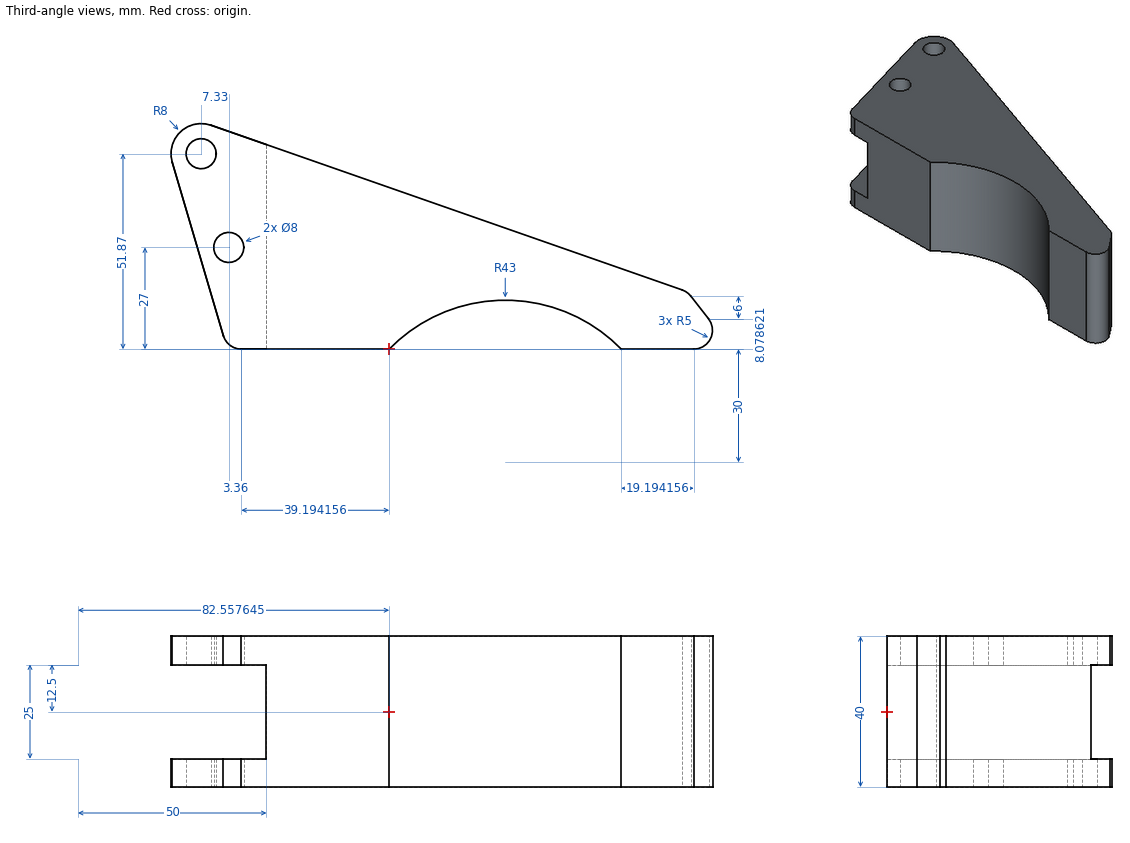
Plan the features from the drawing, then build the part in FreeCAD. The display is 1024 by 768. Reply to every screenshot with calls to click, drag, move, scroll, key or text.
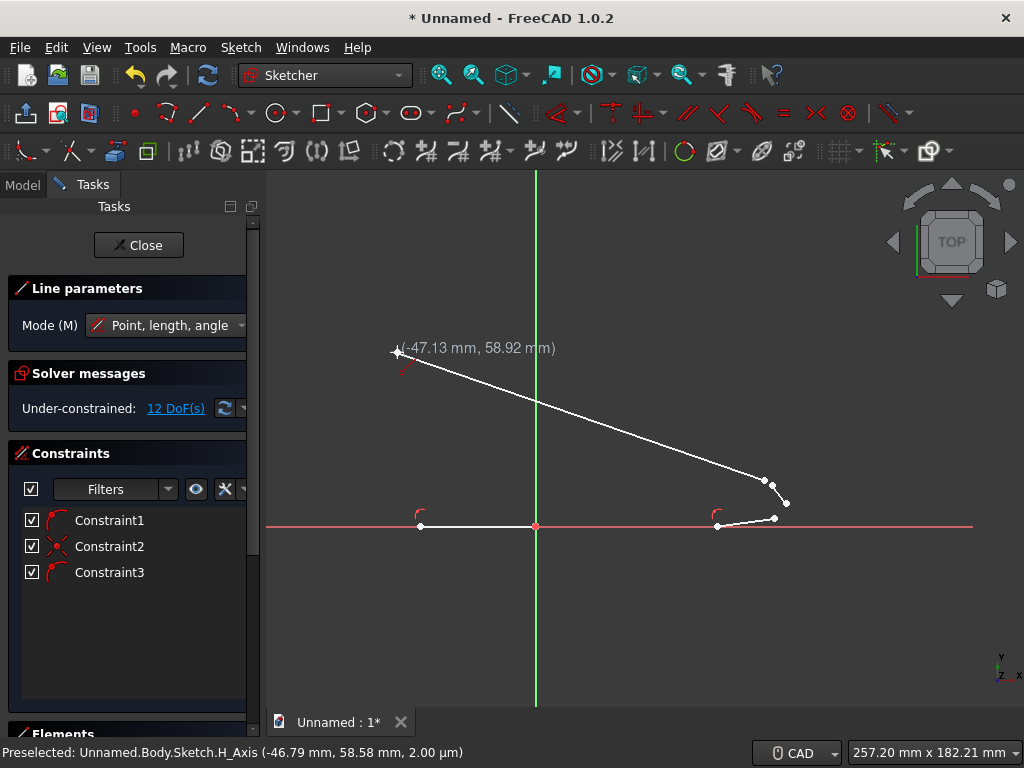
click(366, 380)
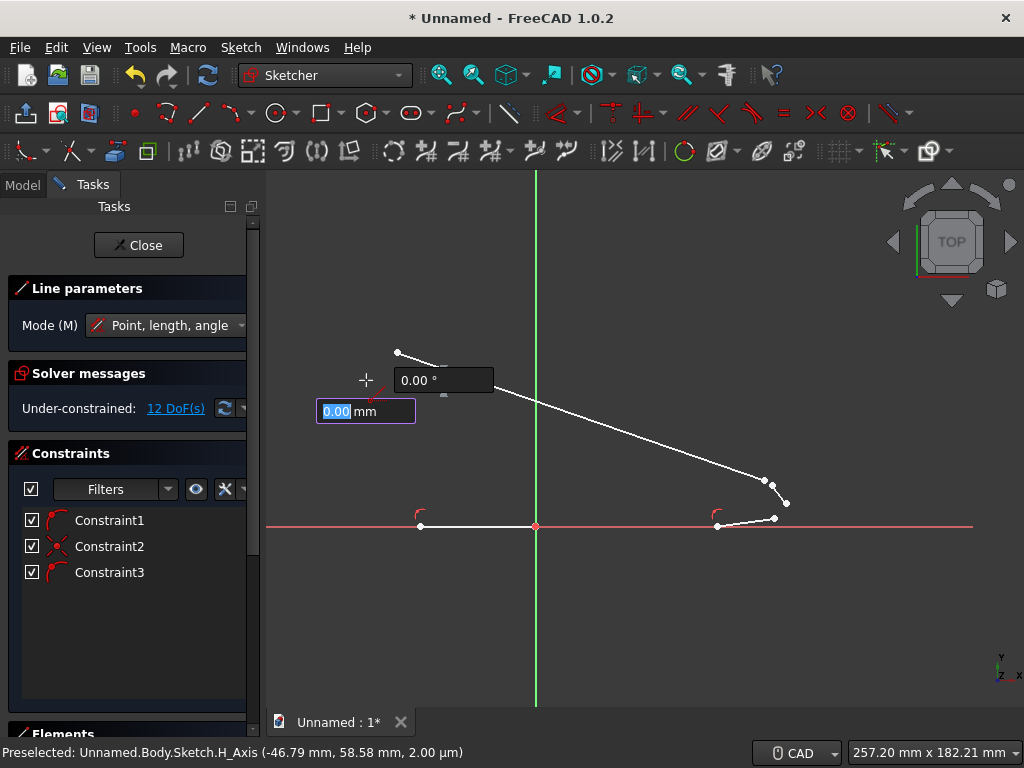
scroll(406, 516, up, 3)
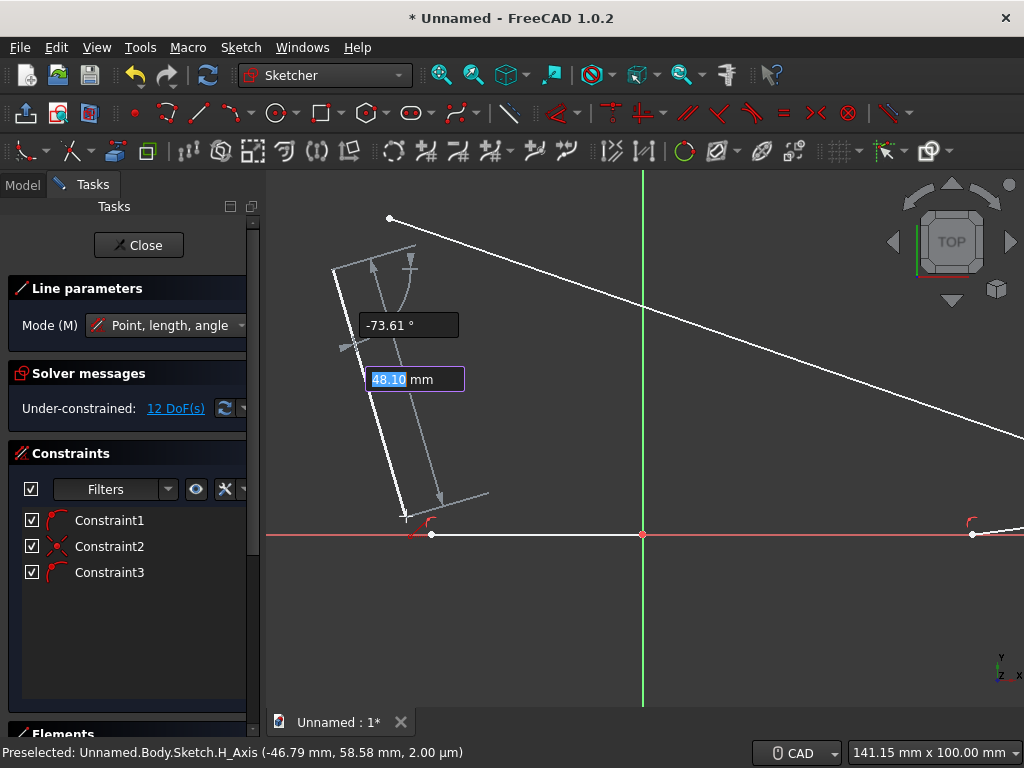
click(406, 516)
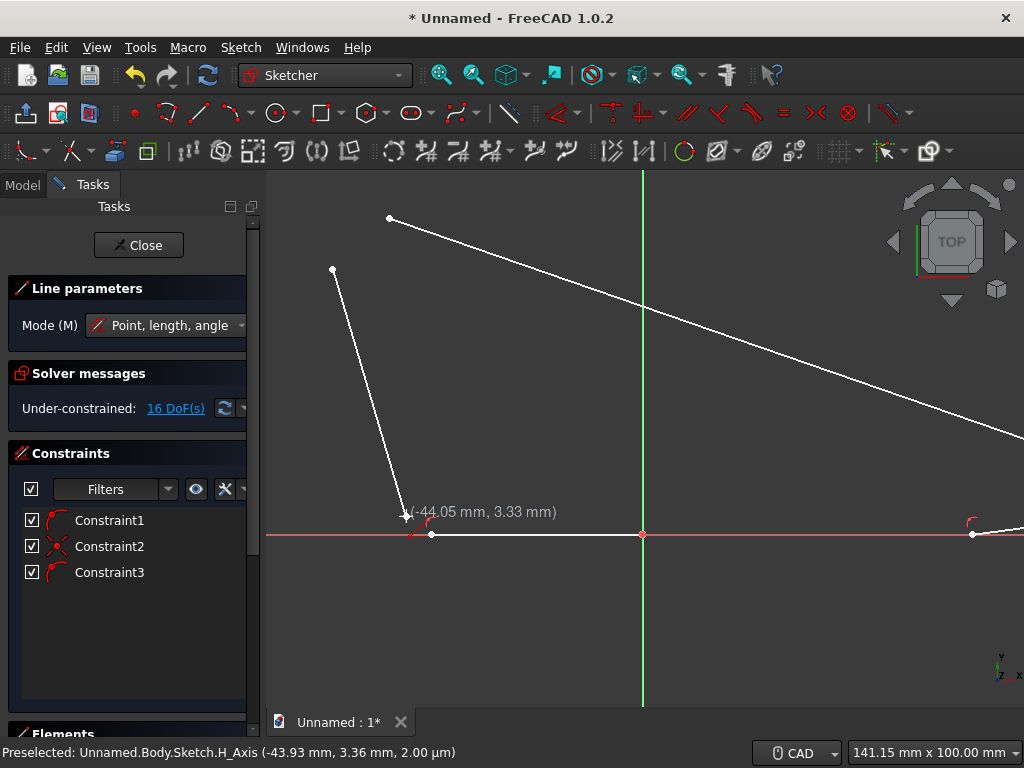
click(232, 114)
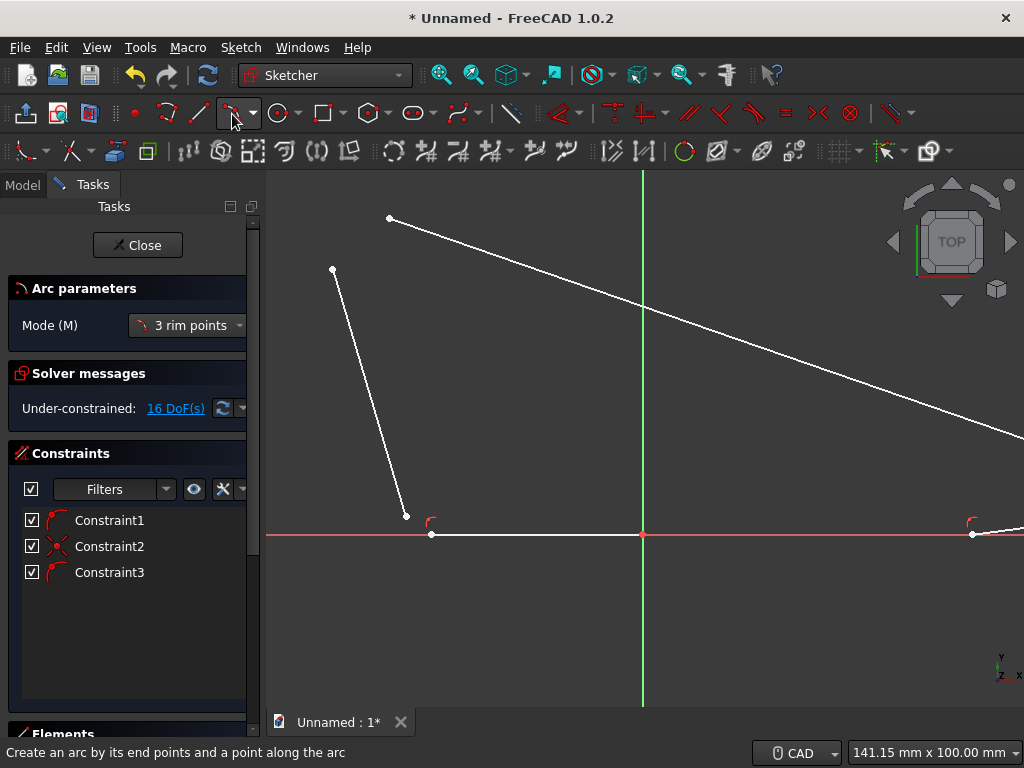
click(643, 535)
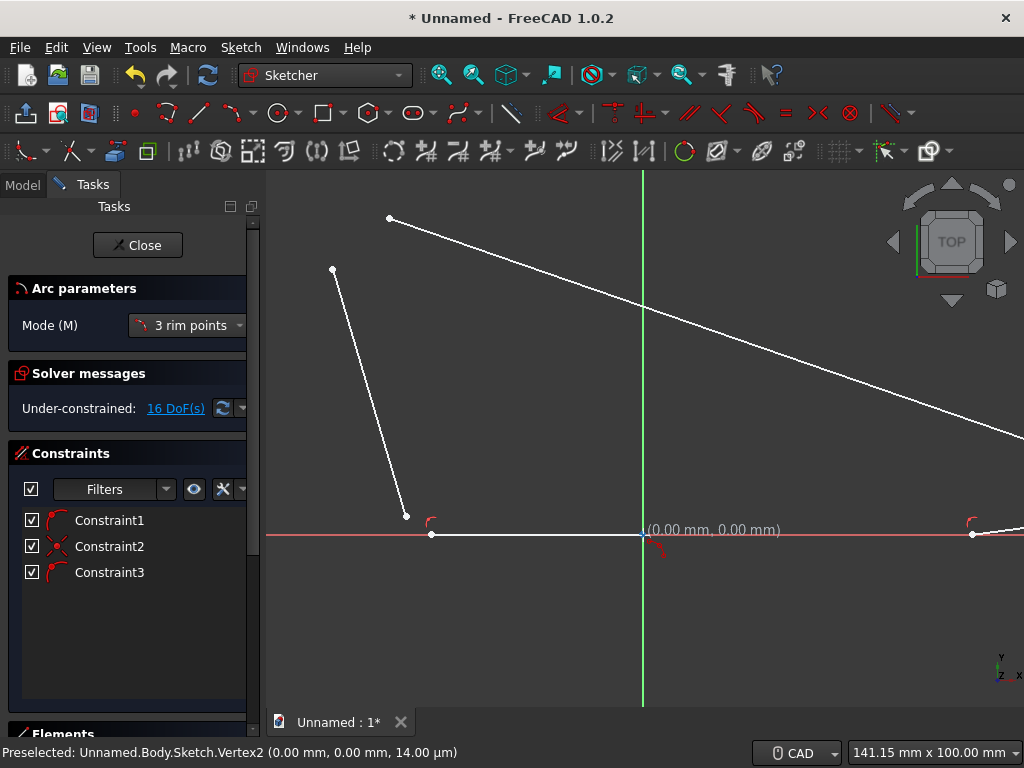
scroll(406, 515, down, 3)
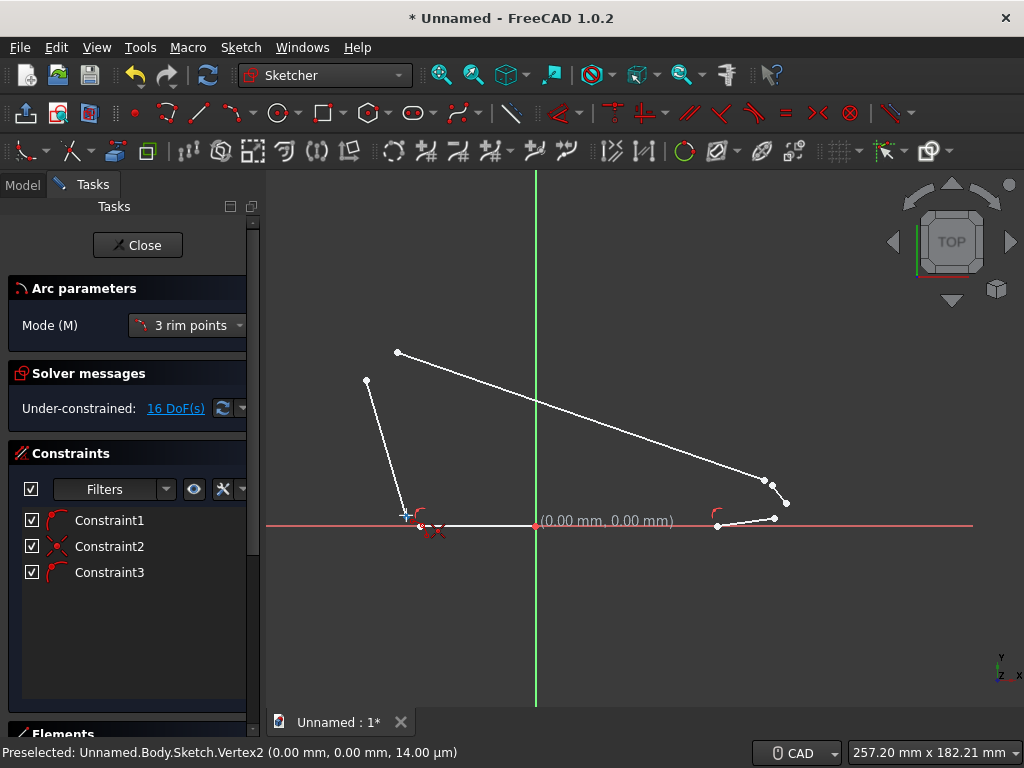
click(717, 526)
click(627, 488)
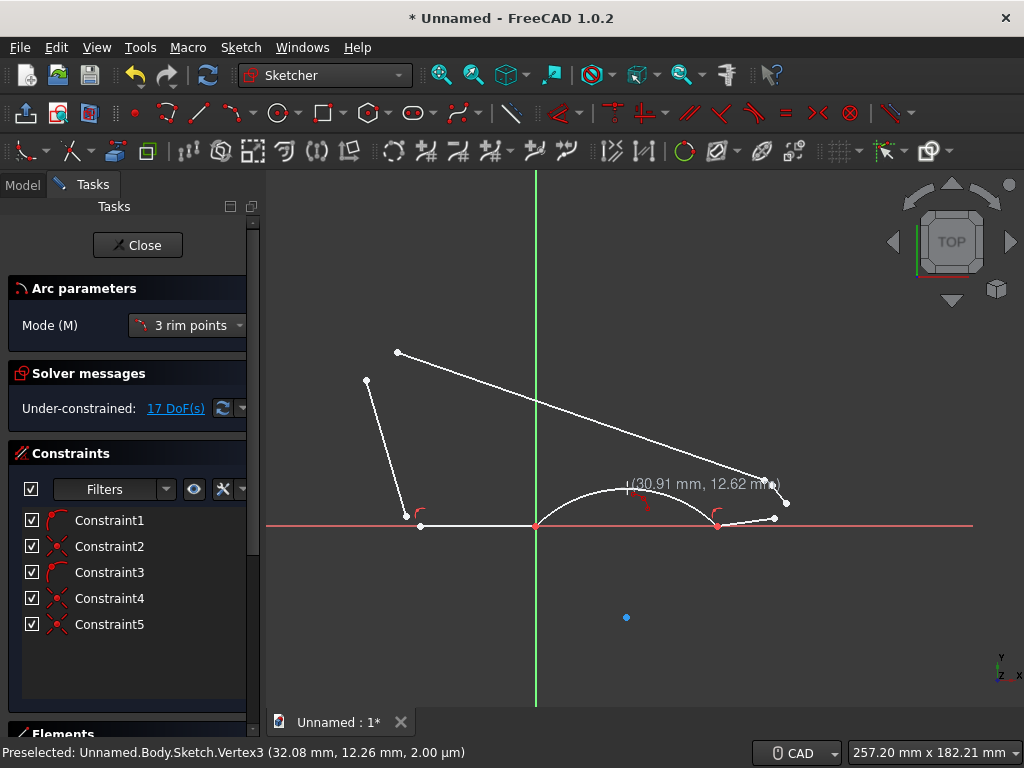
click(774, 519)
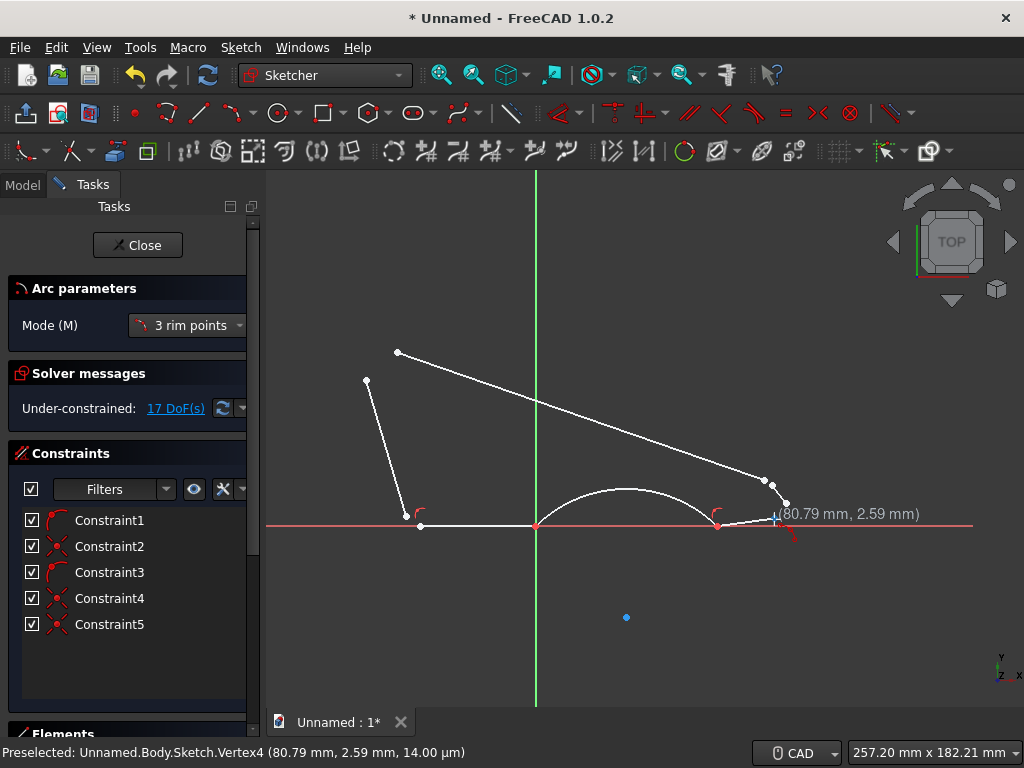
scroll(786, 502, up, 2)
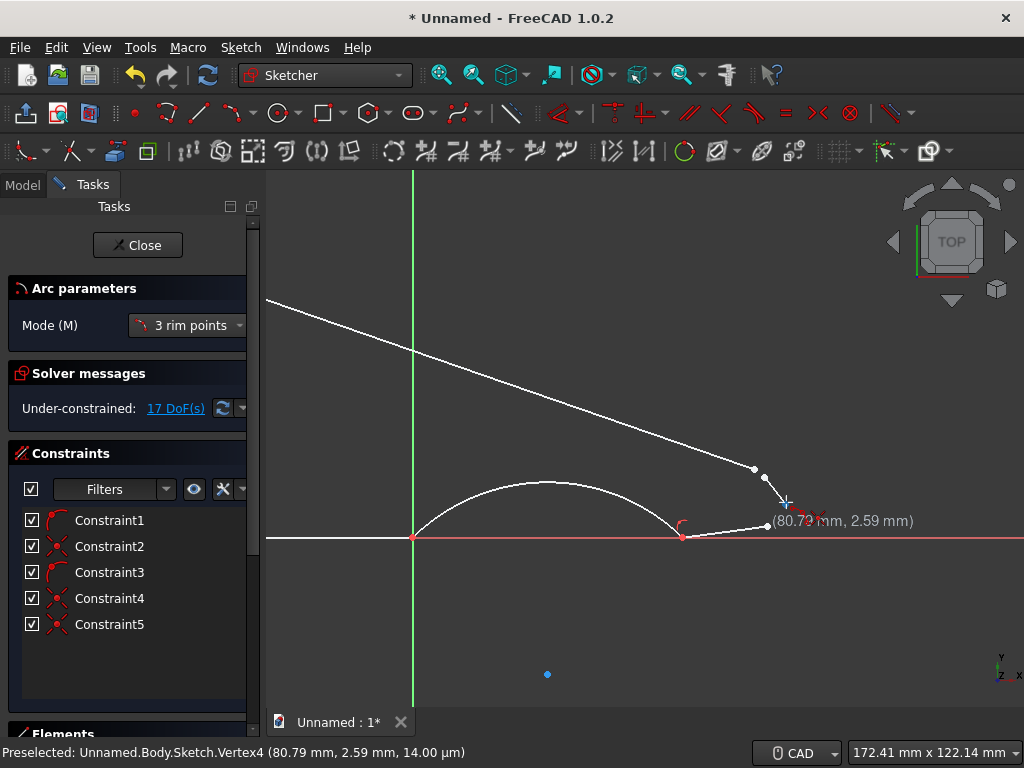
click(786, 504)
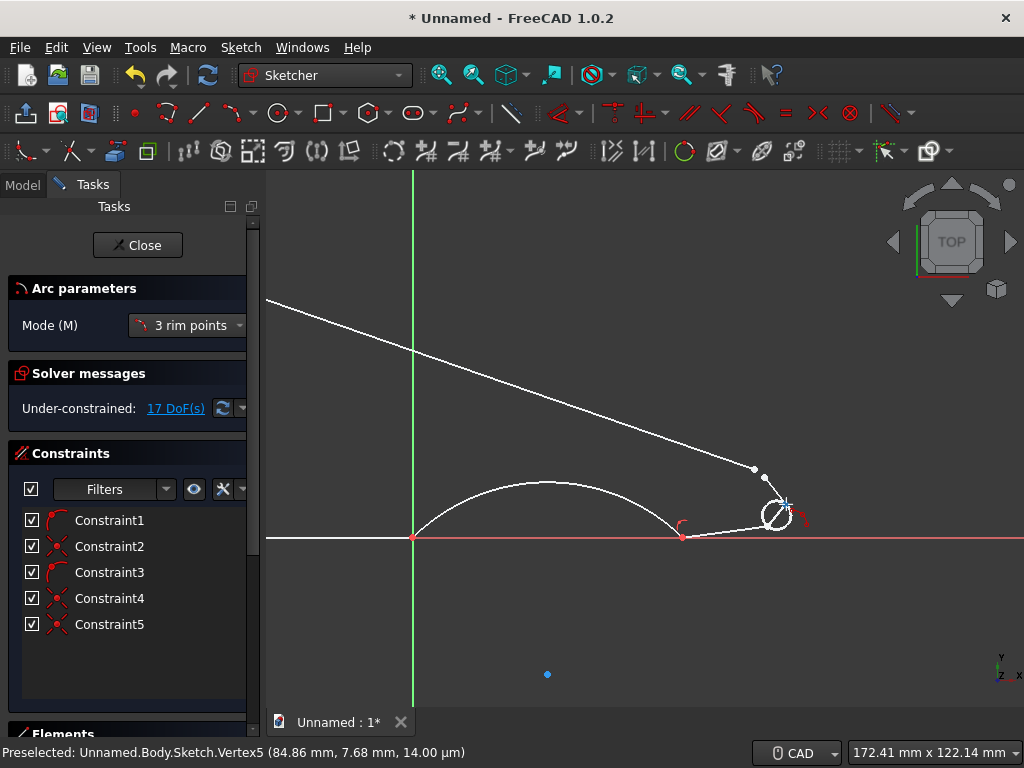
scroll(788, 525, up, 2)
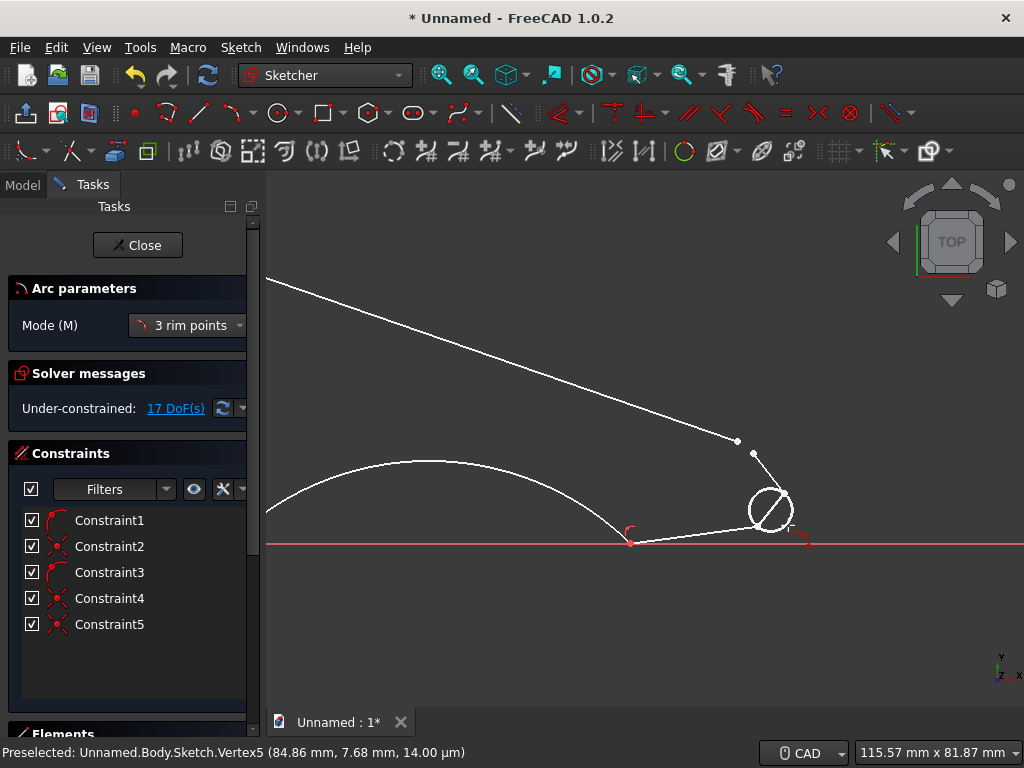
click(787, 525)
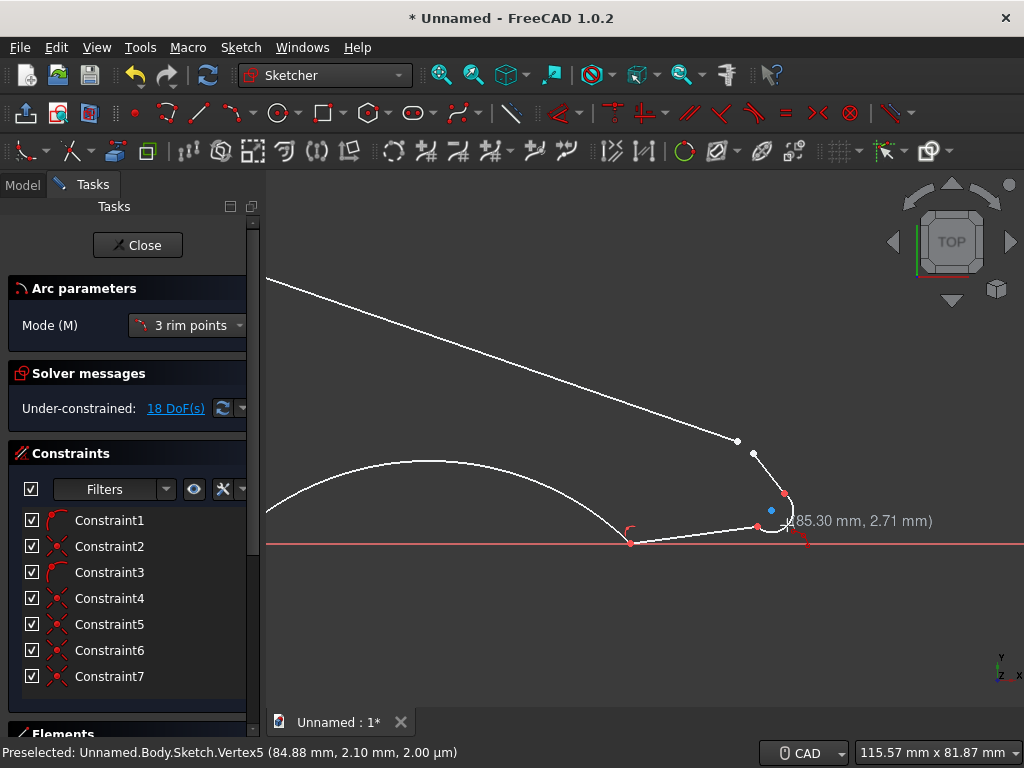
click(753, 453)
click(737, 442)